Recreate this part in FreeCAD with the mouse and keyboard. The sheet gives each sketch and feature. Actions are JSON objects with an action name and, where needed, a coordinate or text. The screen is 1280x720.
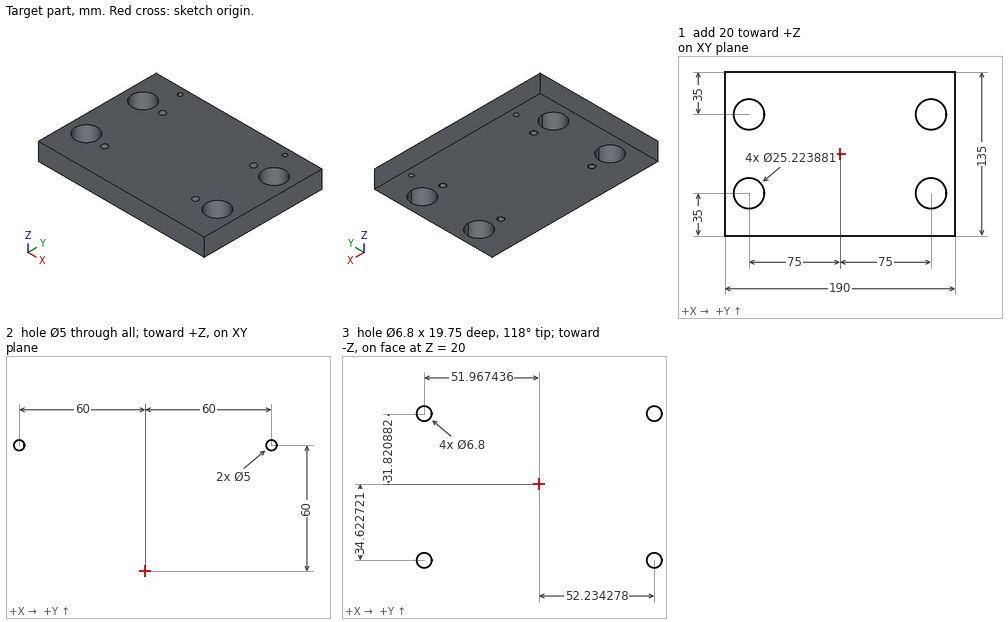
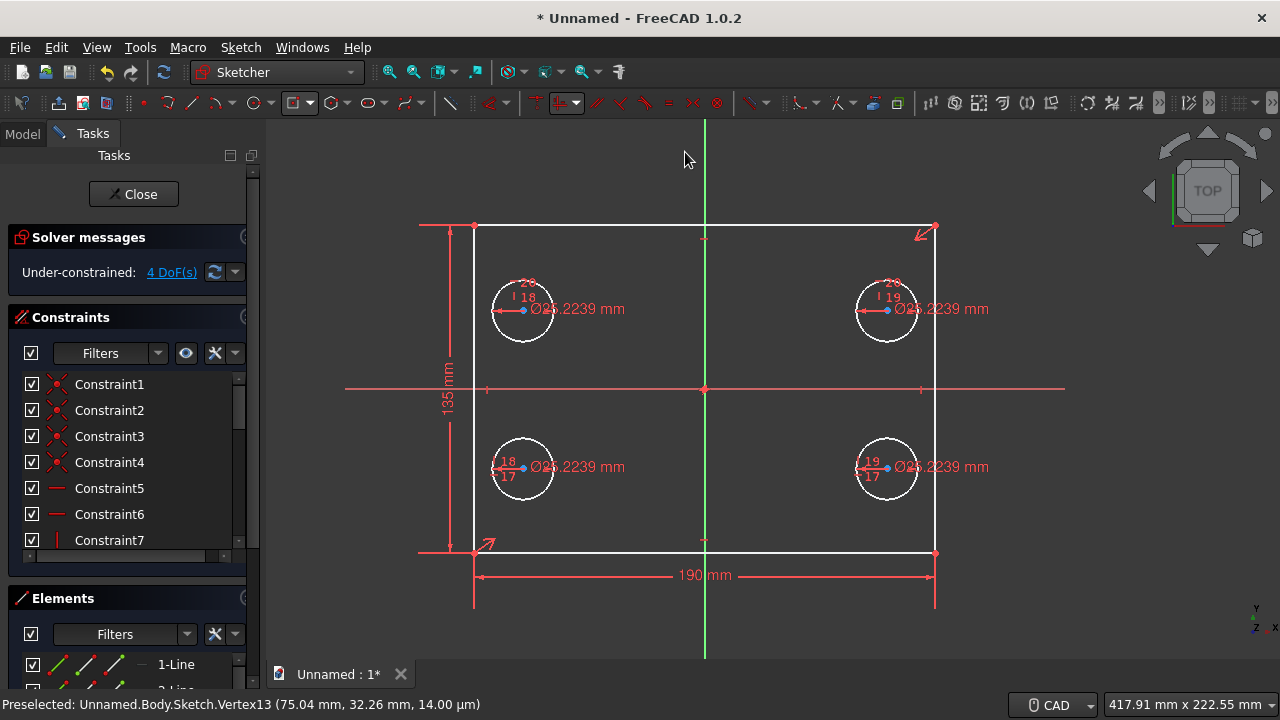
{"action": "left_click", "coordinate": [523, 469]}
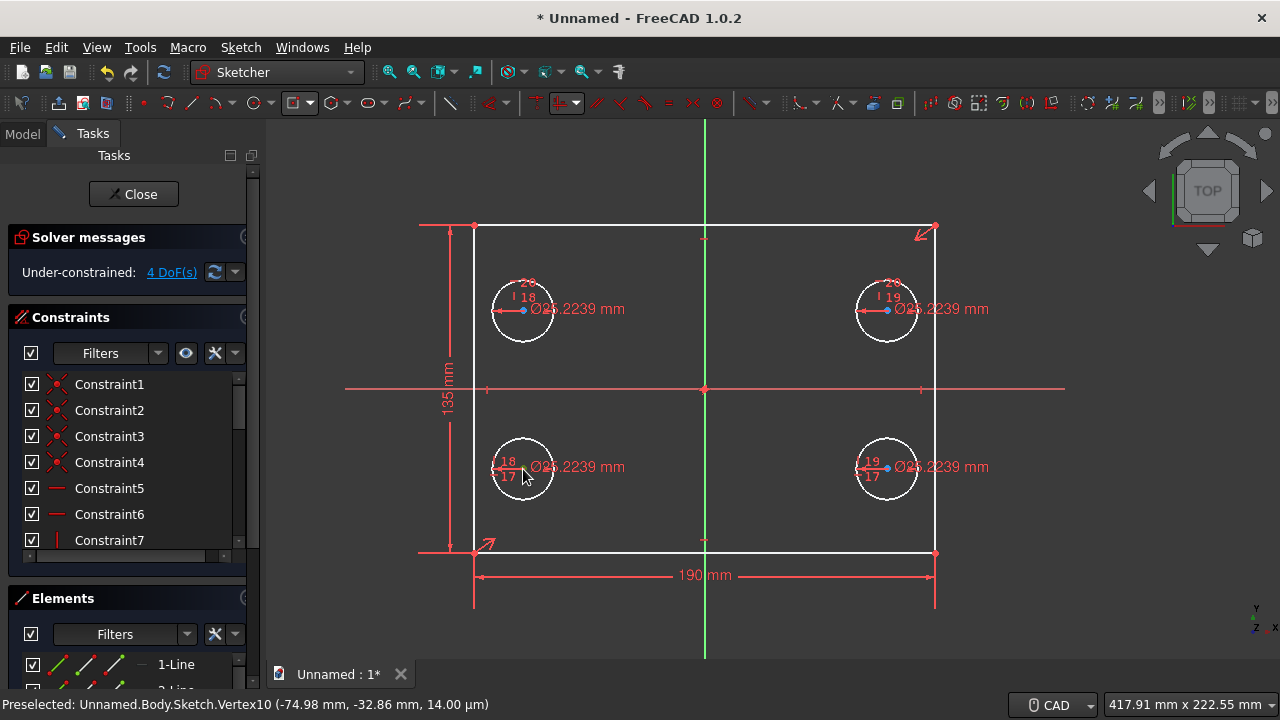
{"action": "key", "text": "l"}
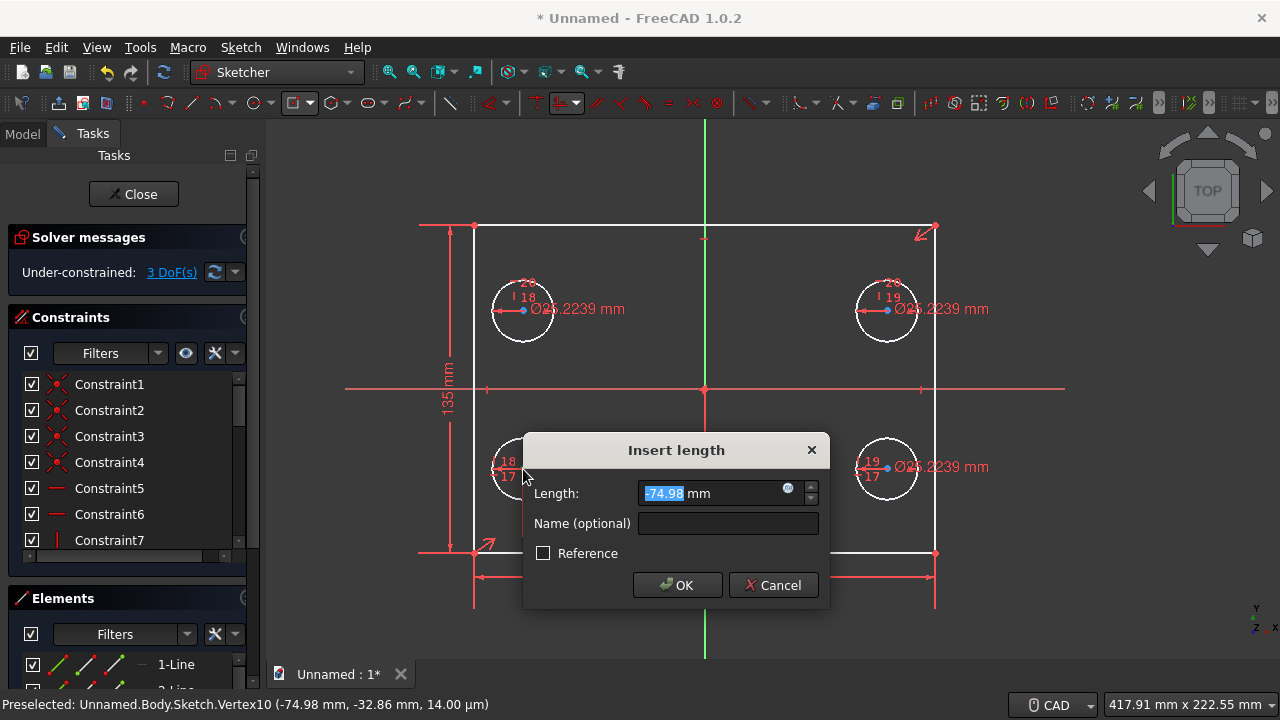
{"action": "type", "text": "-75"}
{"action": "key", "text": "Return"}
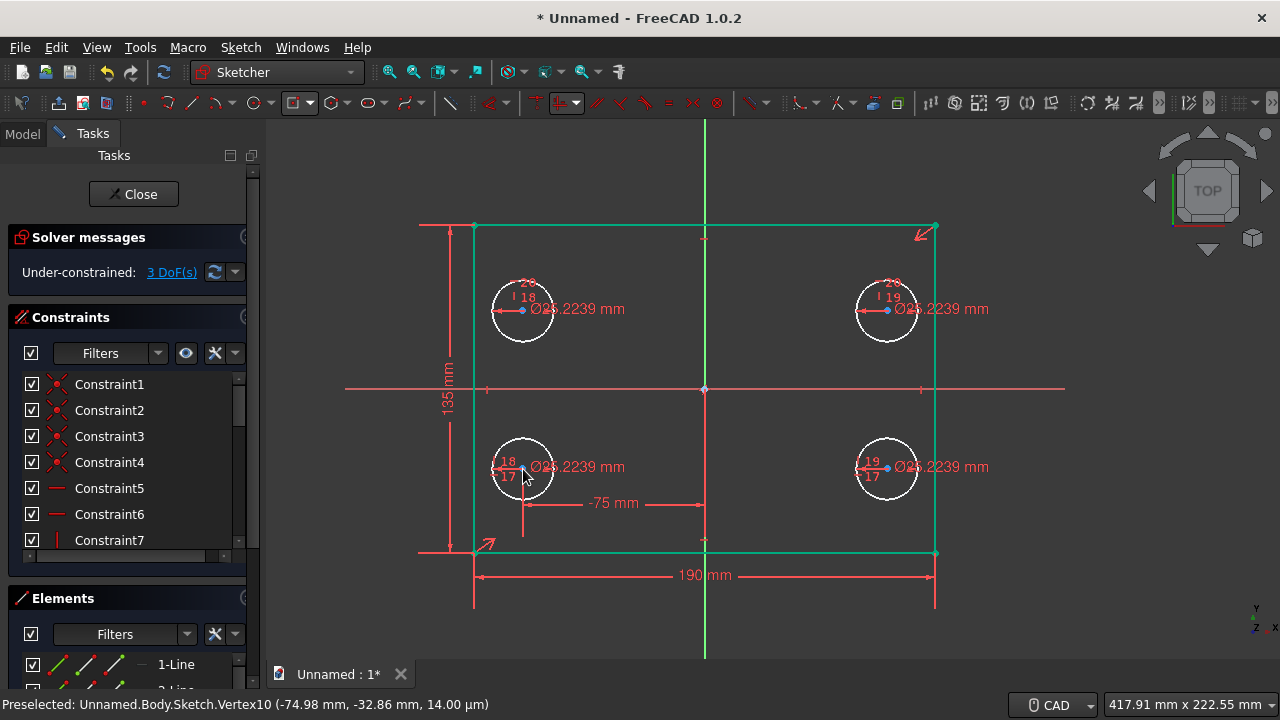
{"action": "left_click", "coordinate": [887, 469]}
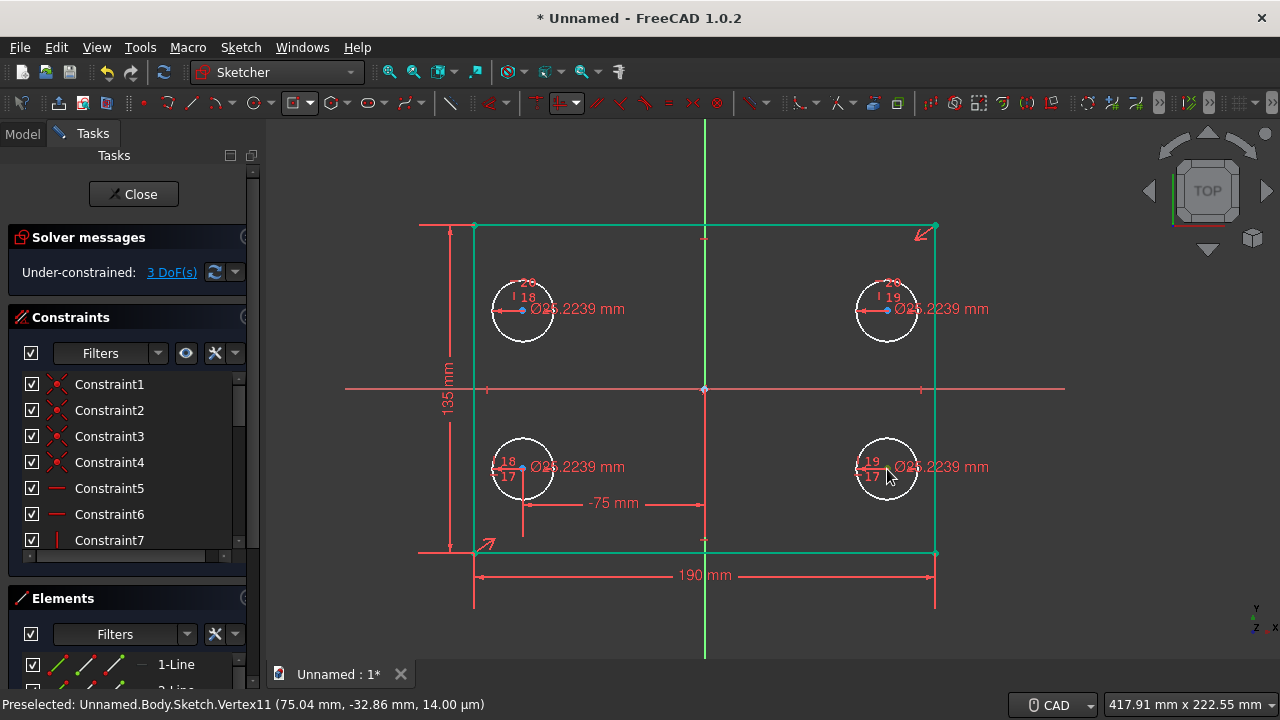
{"action": "key", "text": "l"}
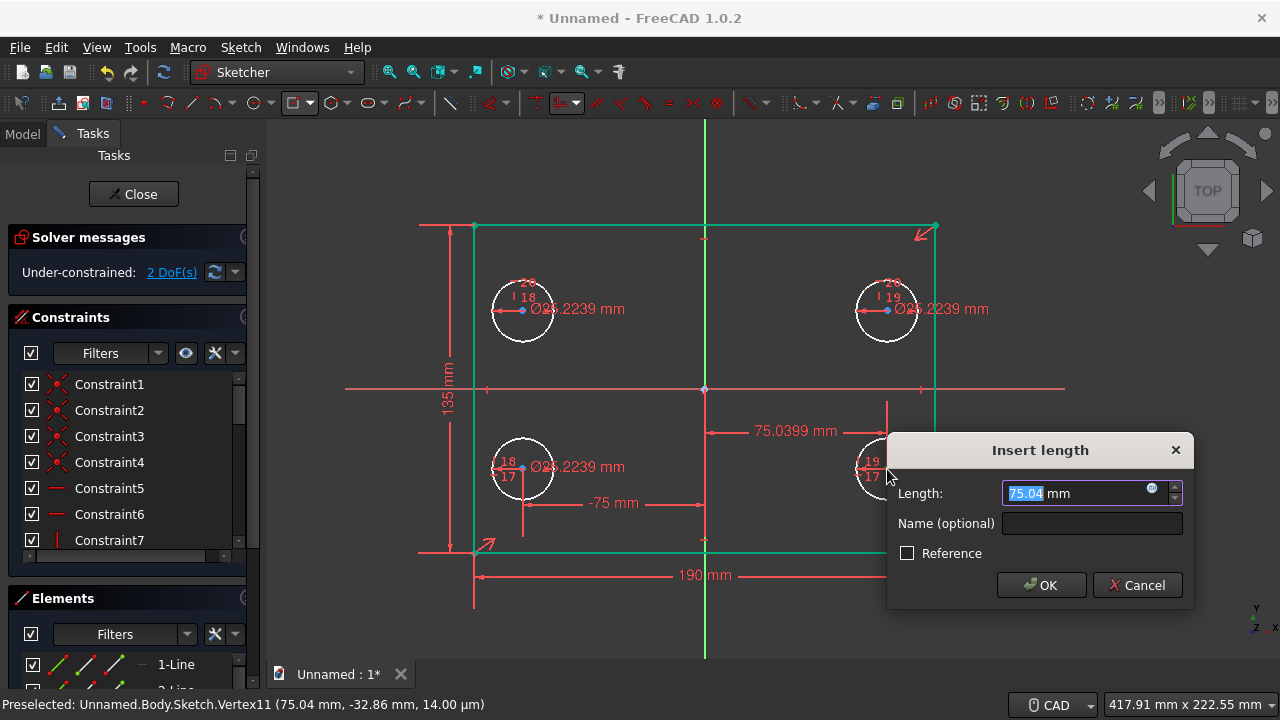
{"action": "type", "text": "75"}
{"action": "key", "text": "Return"}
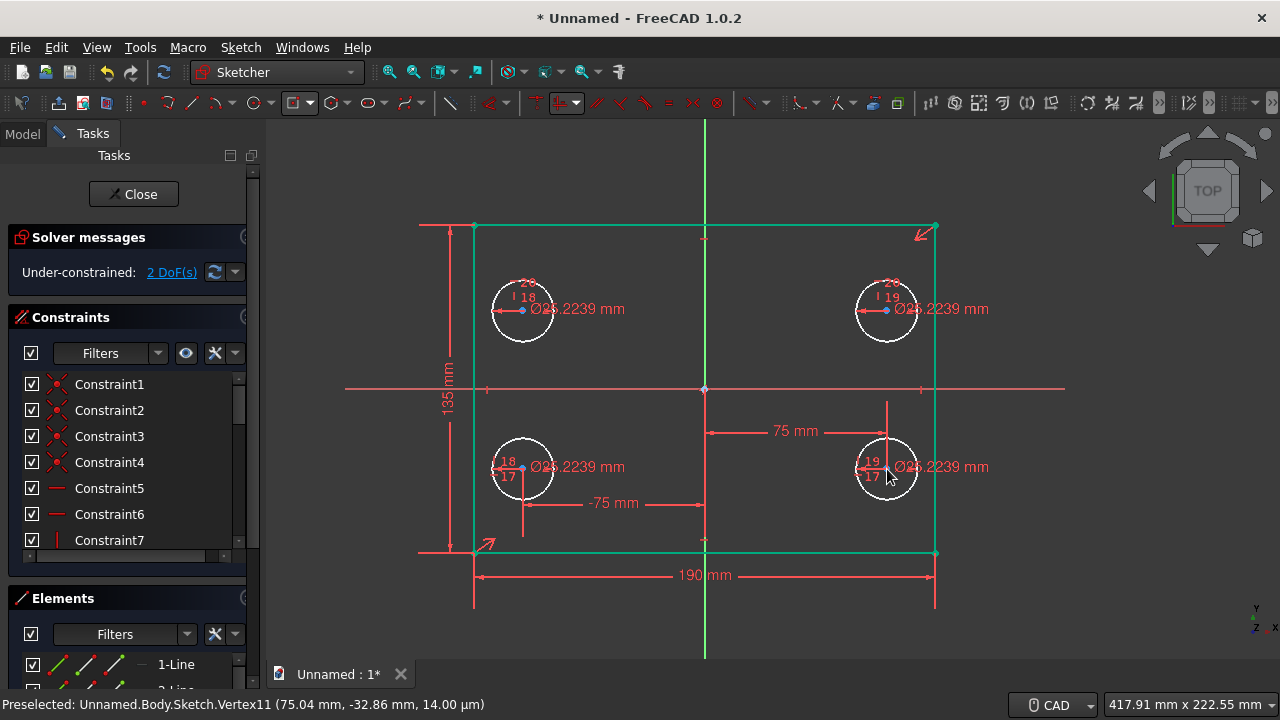
{"action": "left_click", "coordinate": [474, 553]}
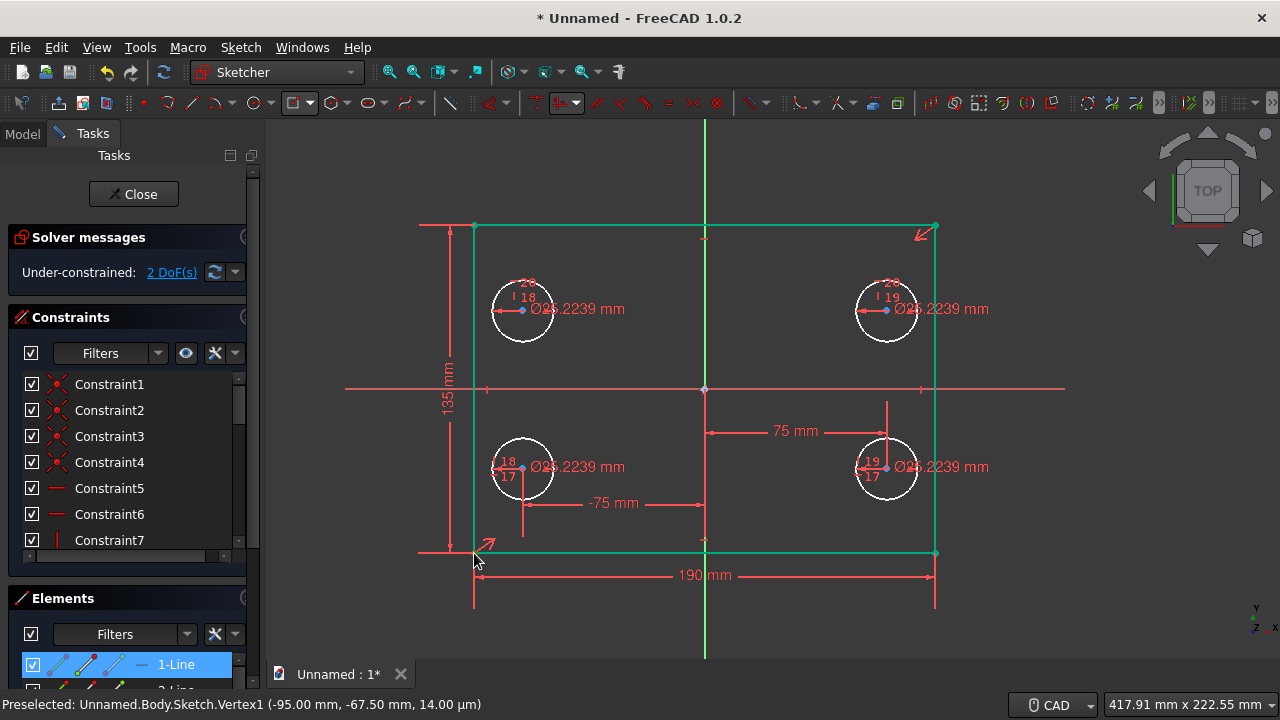
{"action": "left_click", "coordinate": [523, 469]}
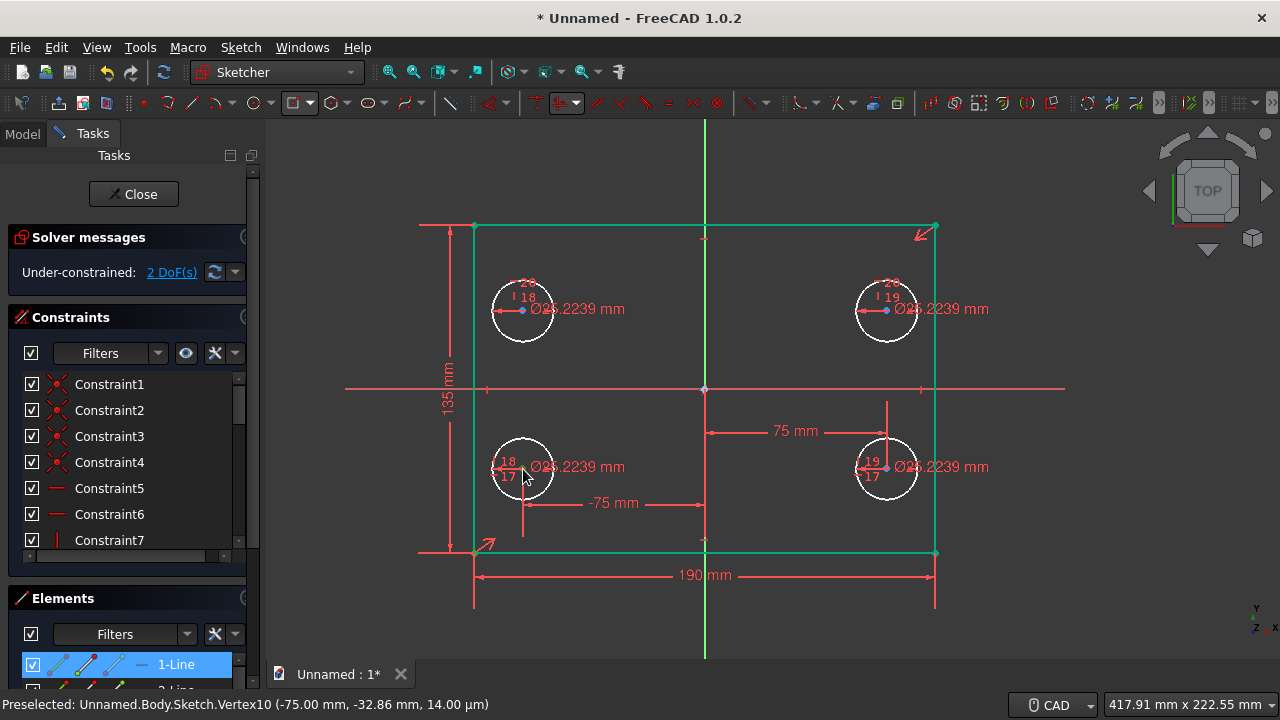
{"action": "left_click", "coordinate": [508, 104]}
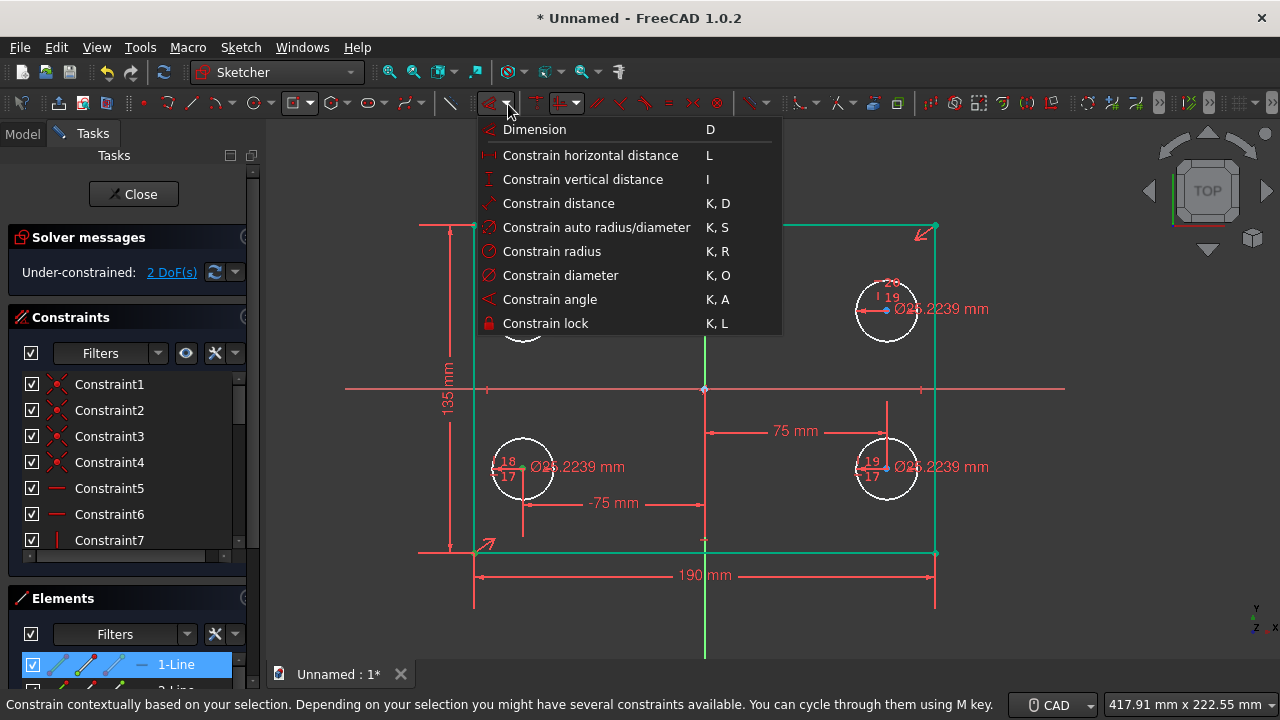
{"action": "left_click", "coordinate": [630, 179]}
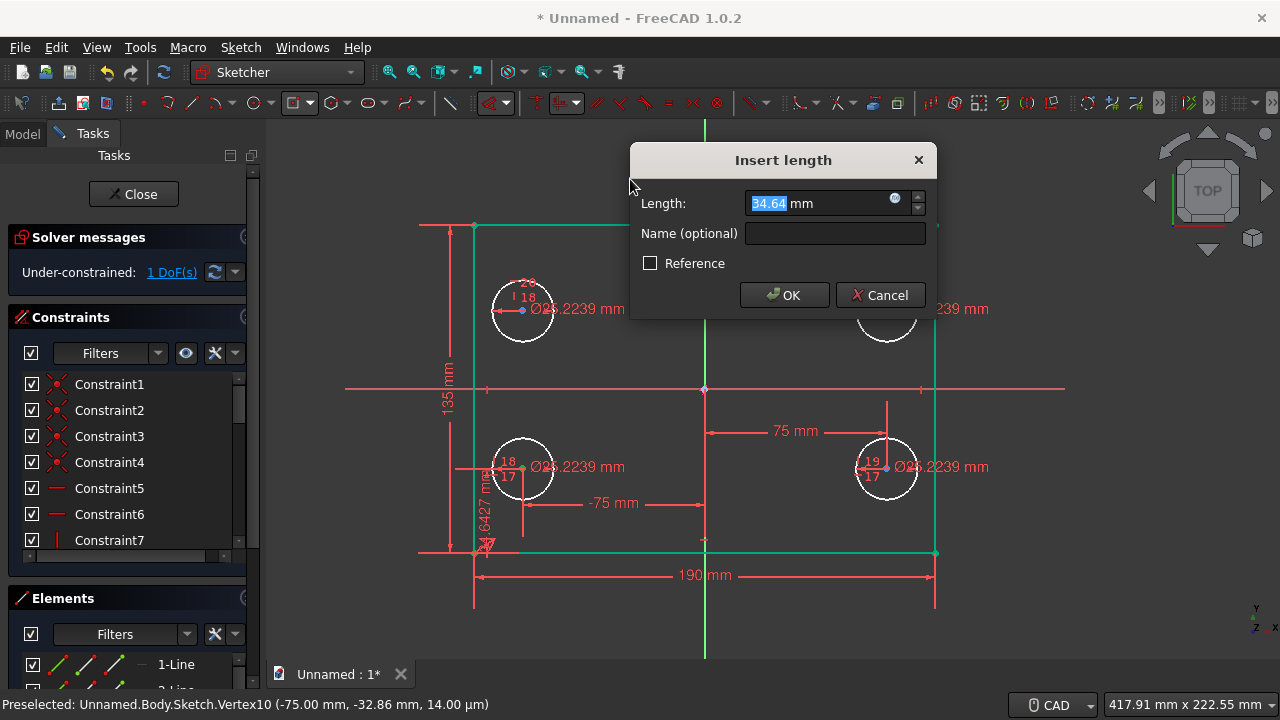
{"action": "type", "text": "35"}
{"action": "key", "text": "Return"}